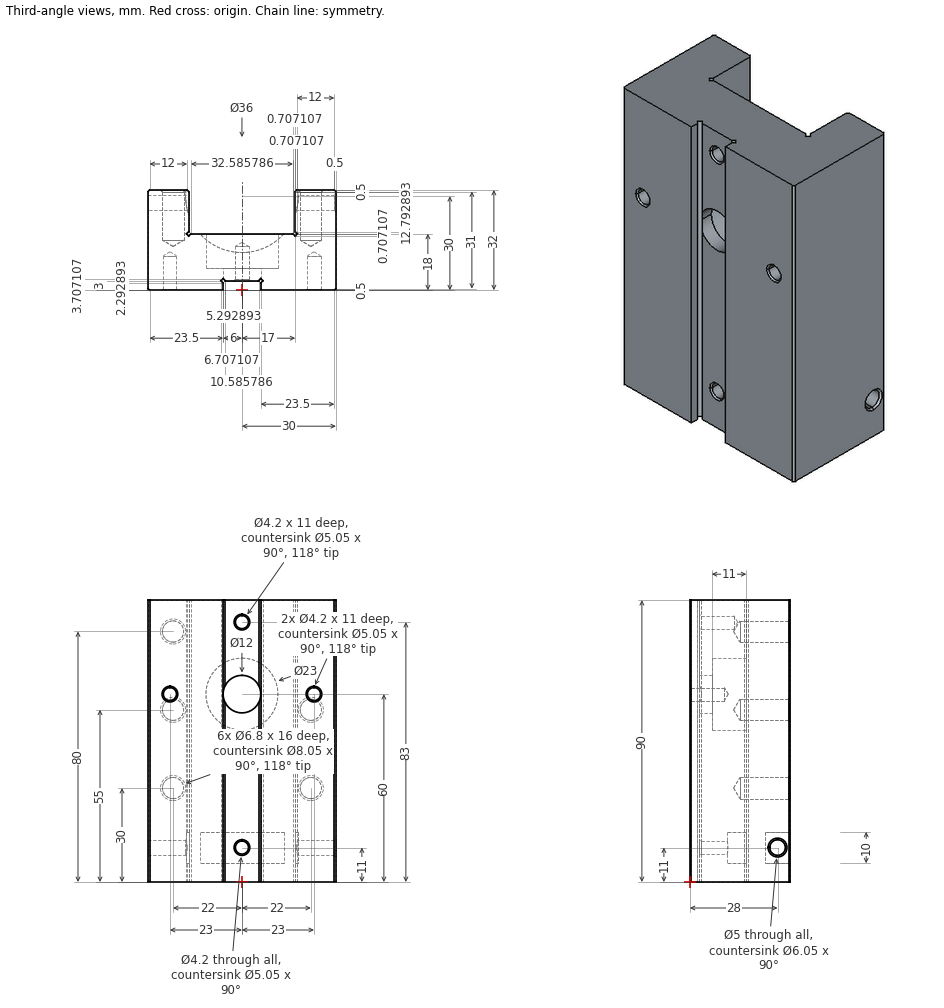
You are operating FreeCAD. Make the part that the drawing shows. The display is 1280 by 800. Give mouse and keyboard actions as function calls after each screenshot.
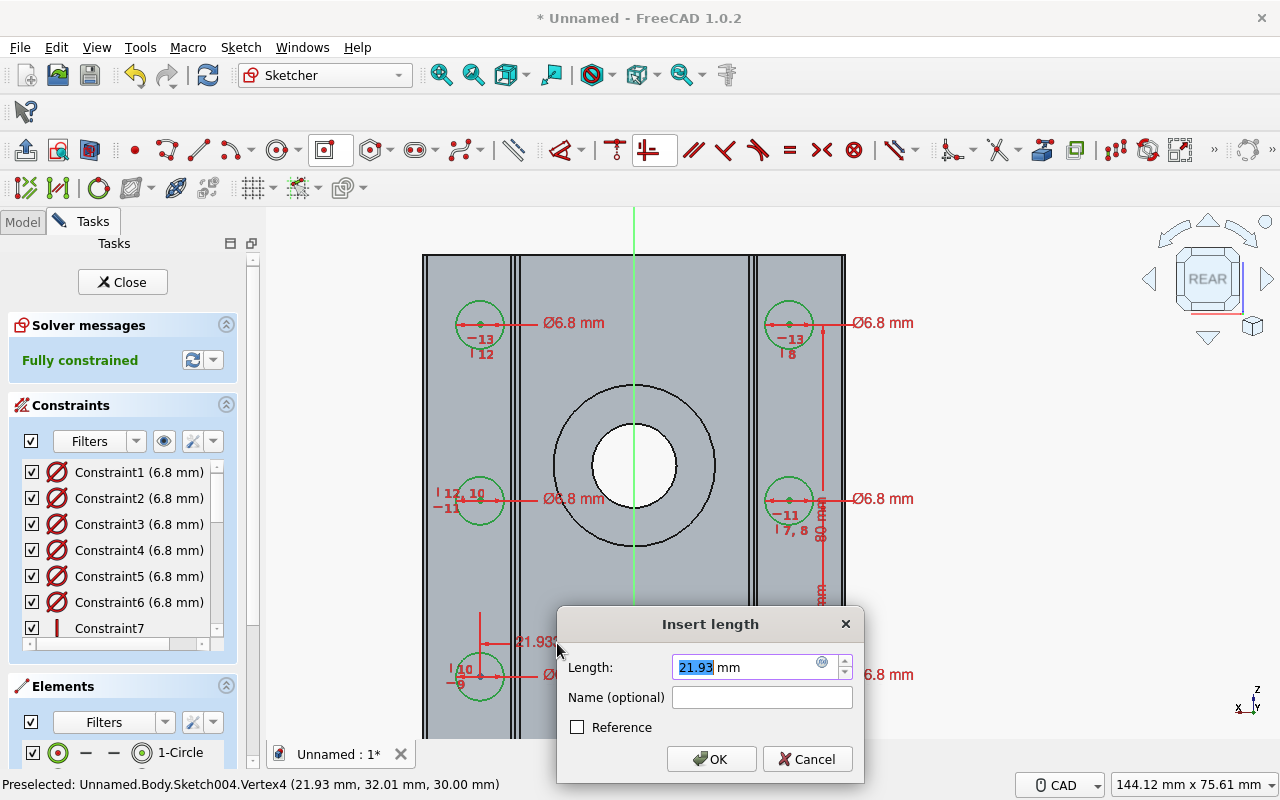
text(22)
key(Return)
key(Escape)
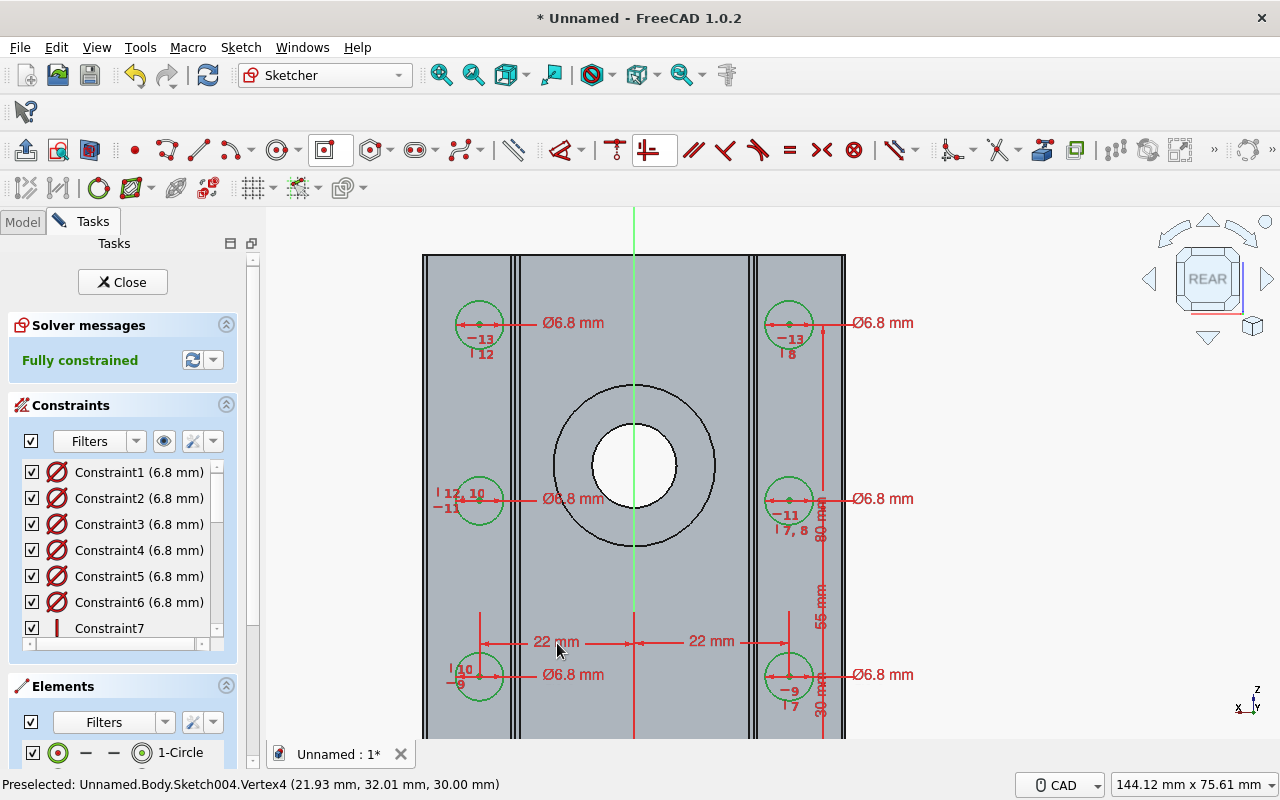
click(123, 282)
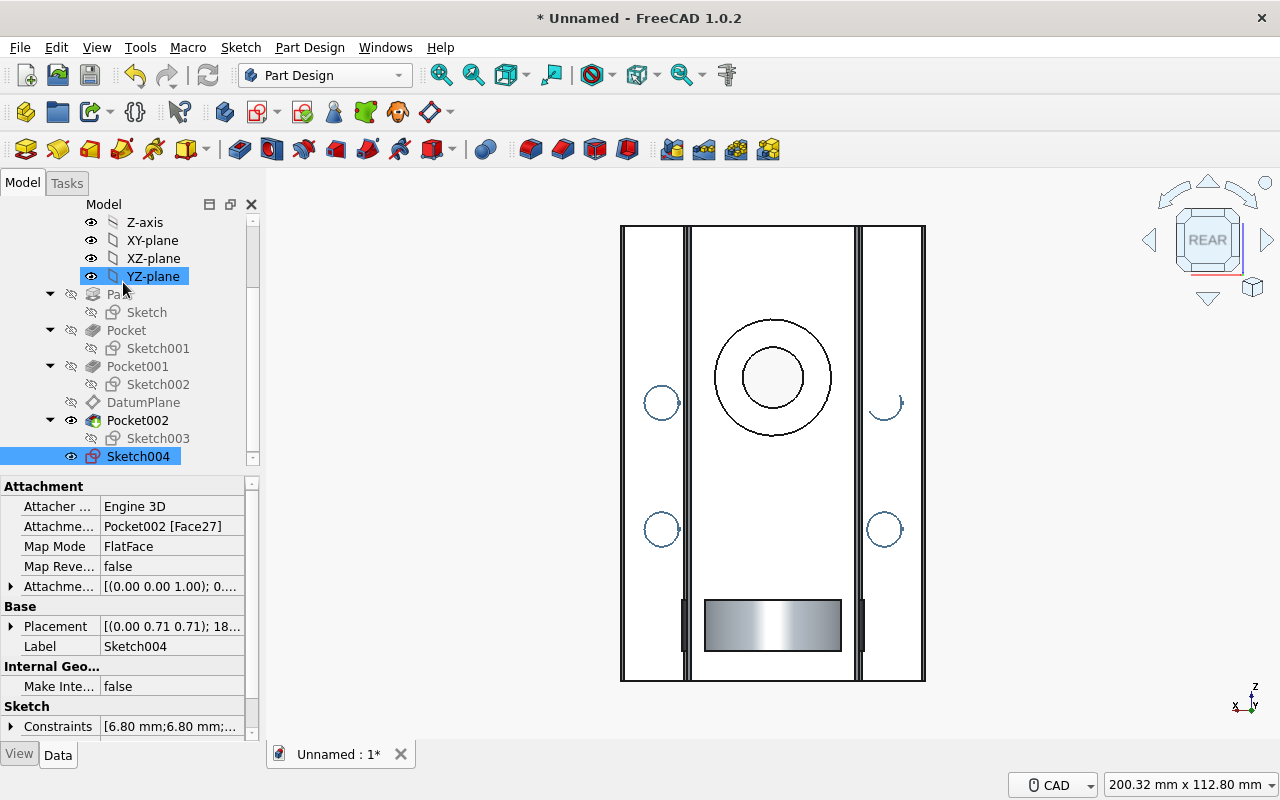
click(272, 150)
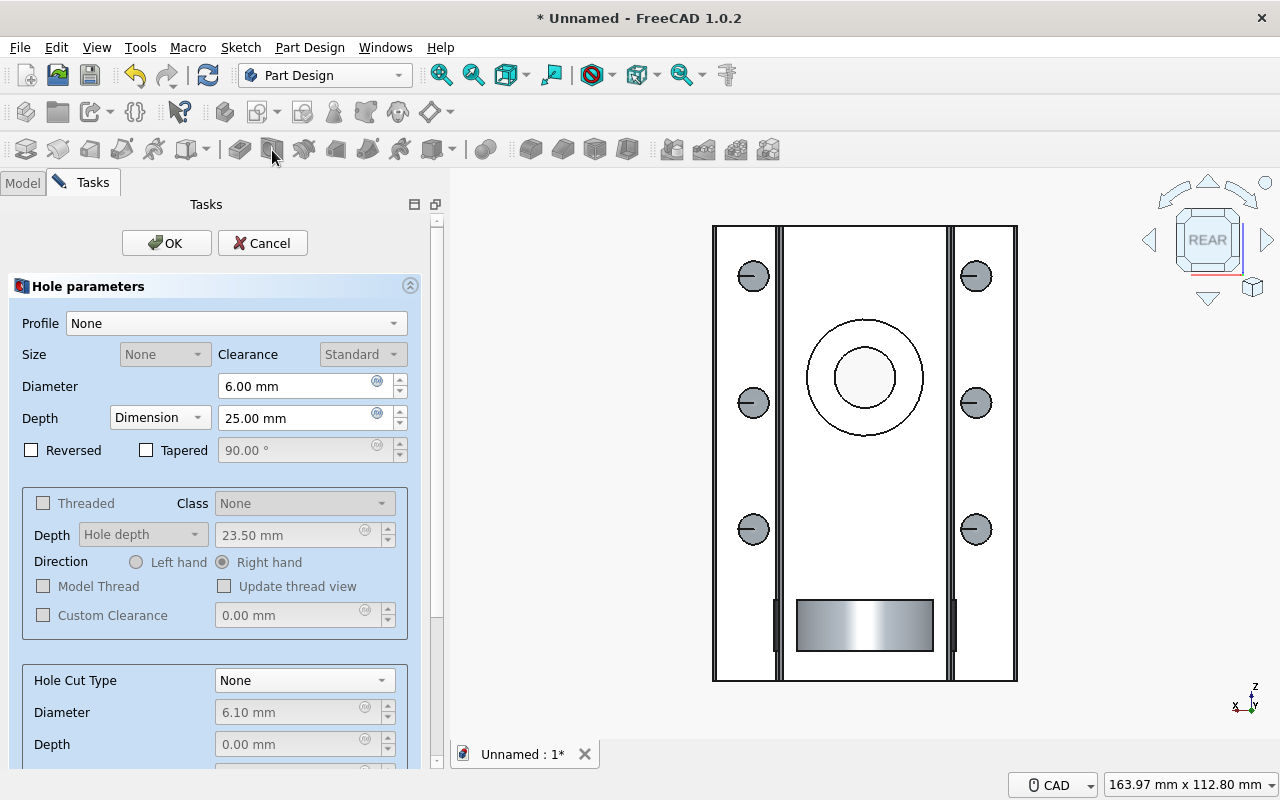
triple_click(305, 386)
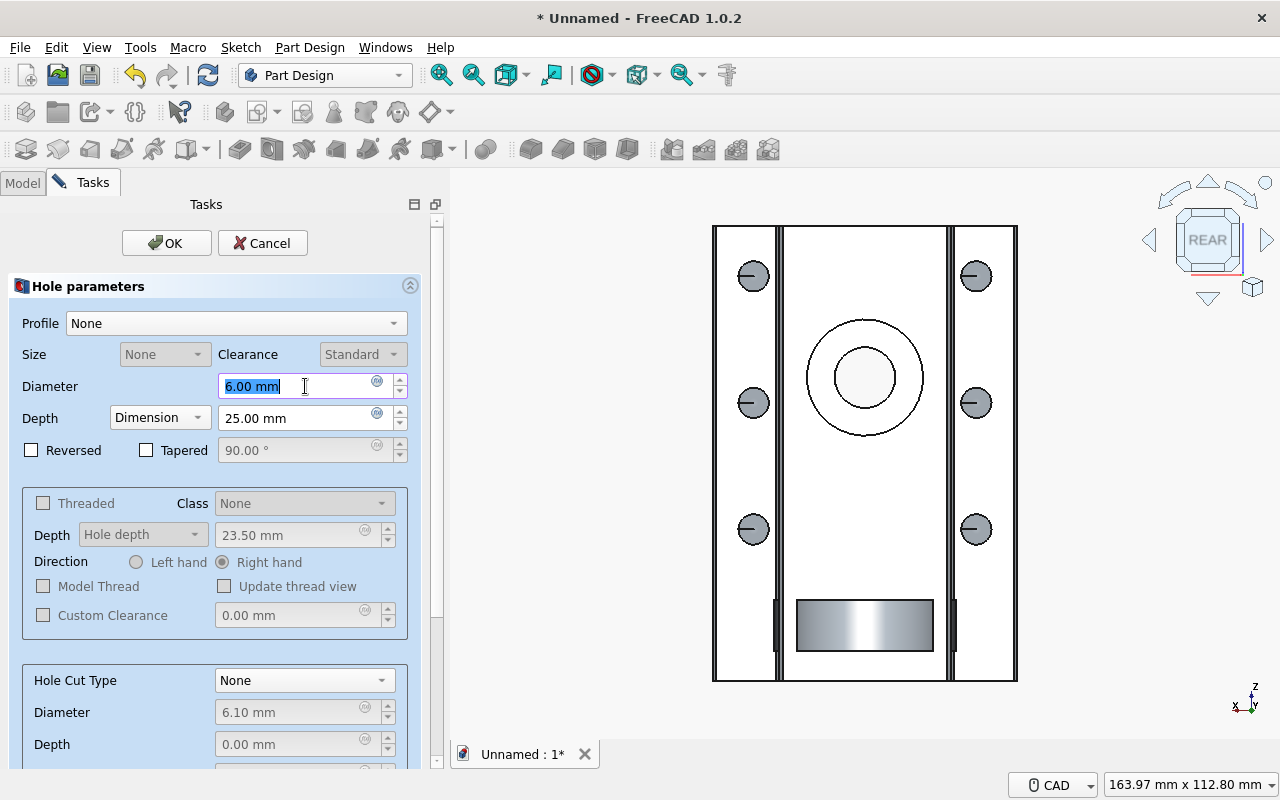
text(6.8)
key(Tab)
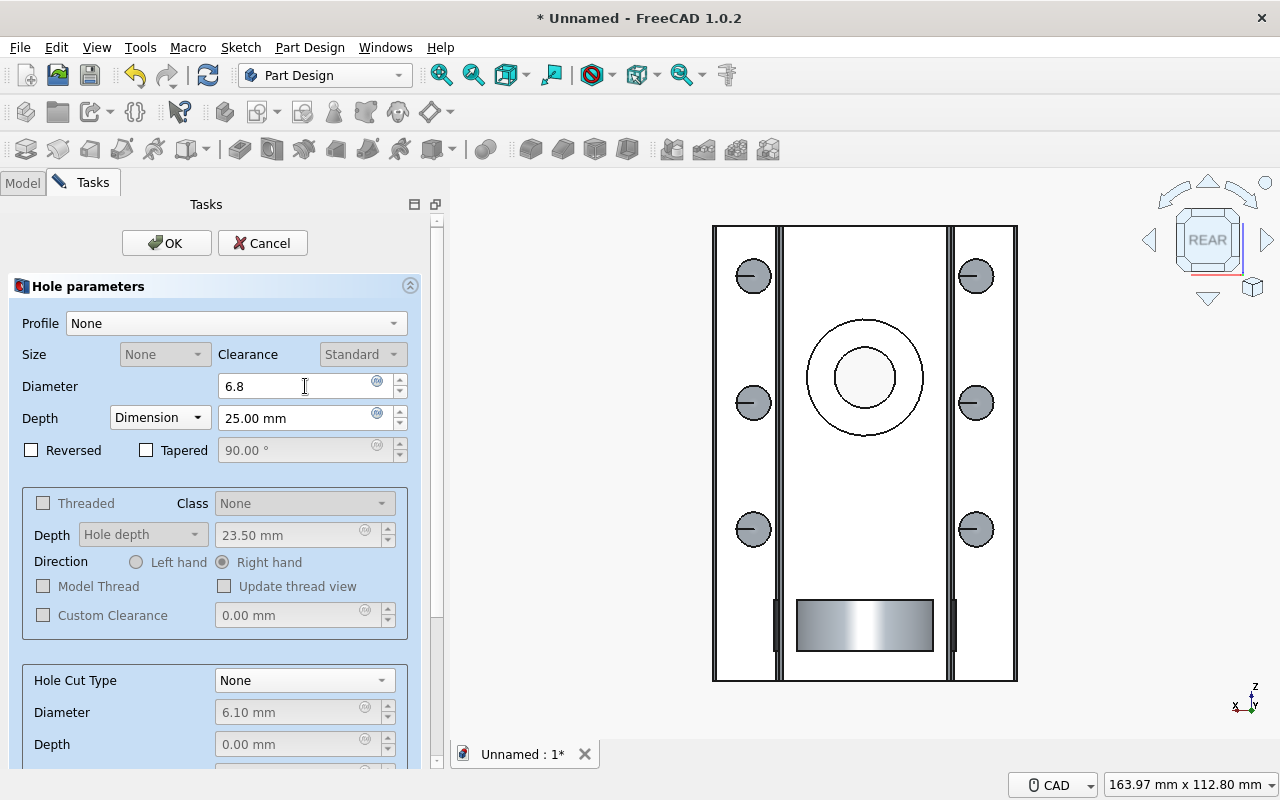
triple_click(305, 418)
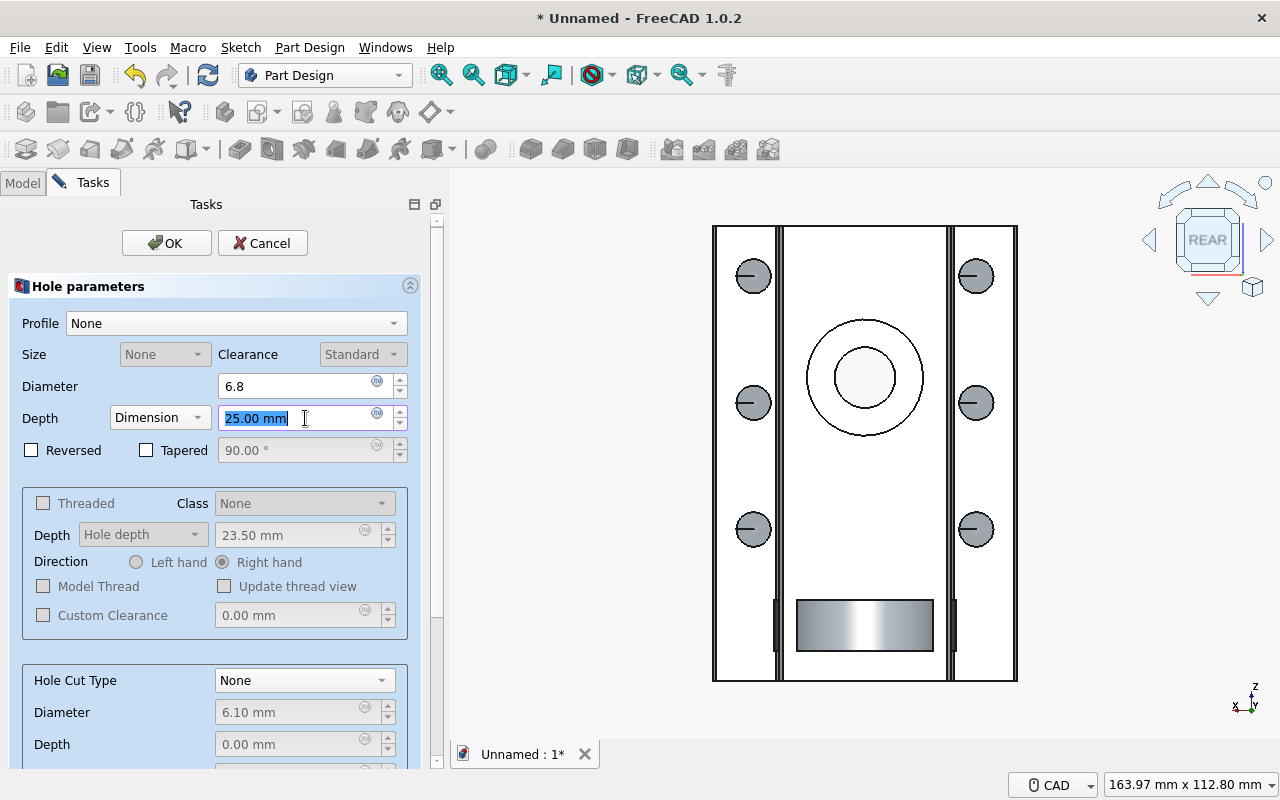
text(16)
key(Tab)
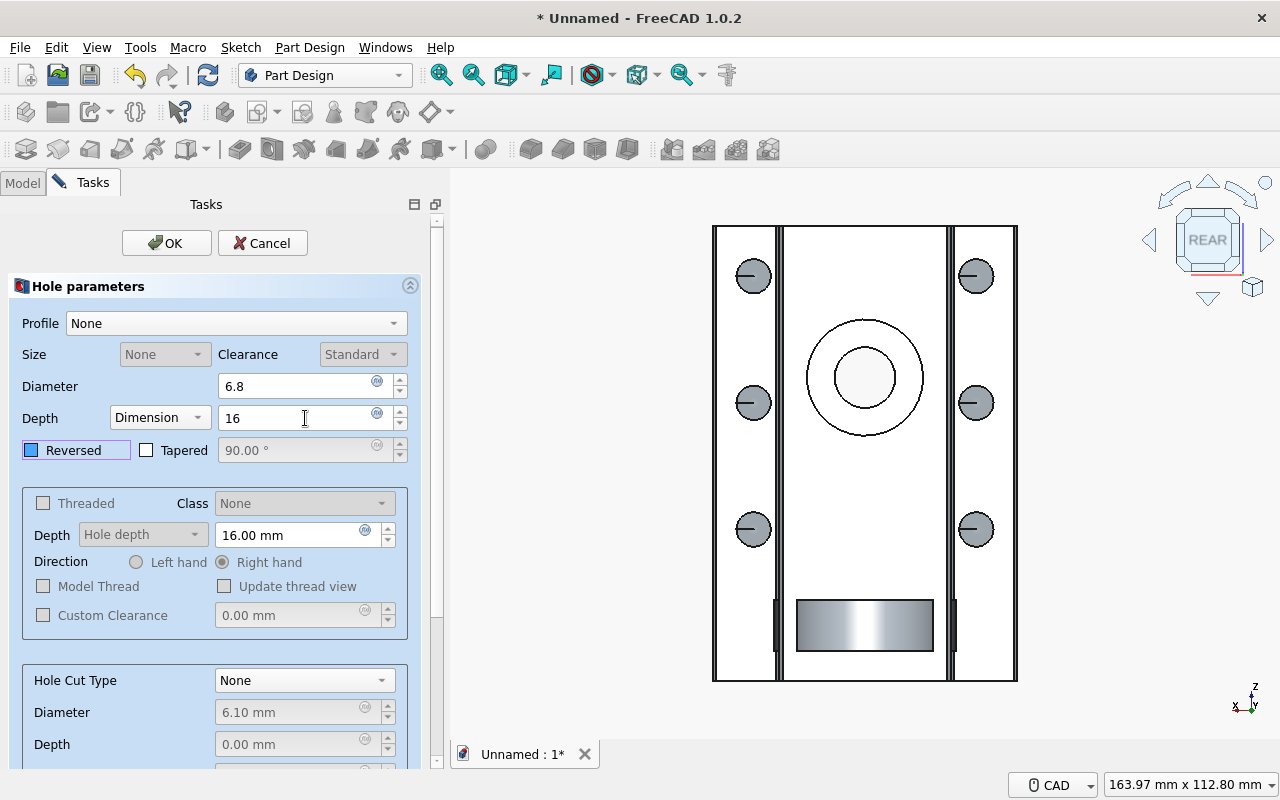
click(306, 680)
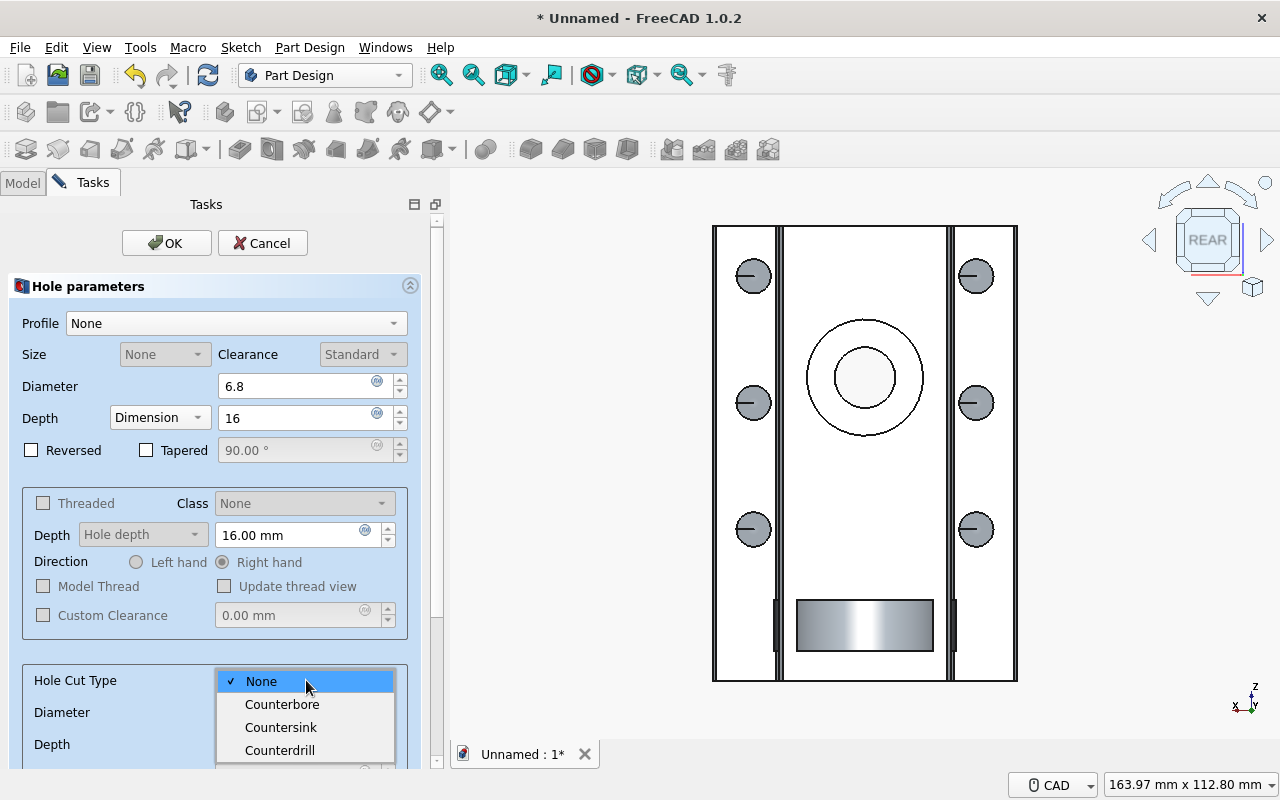
click(304, 728)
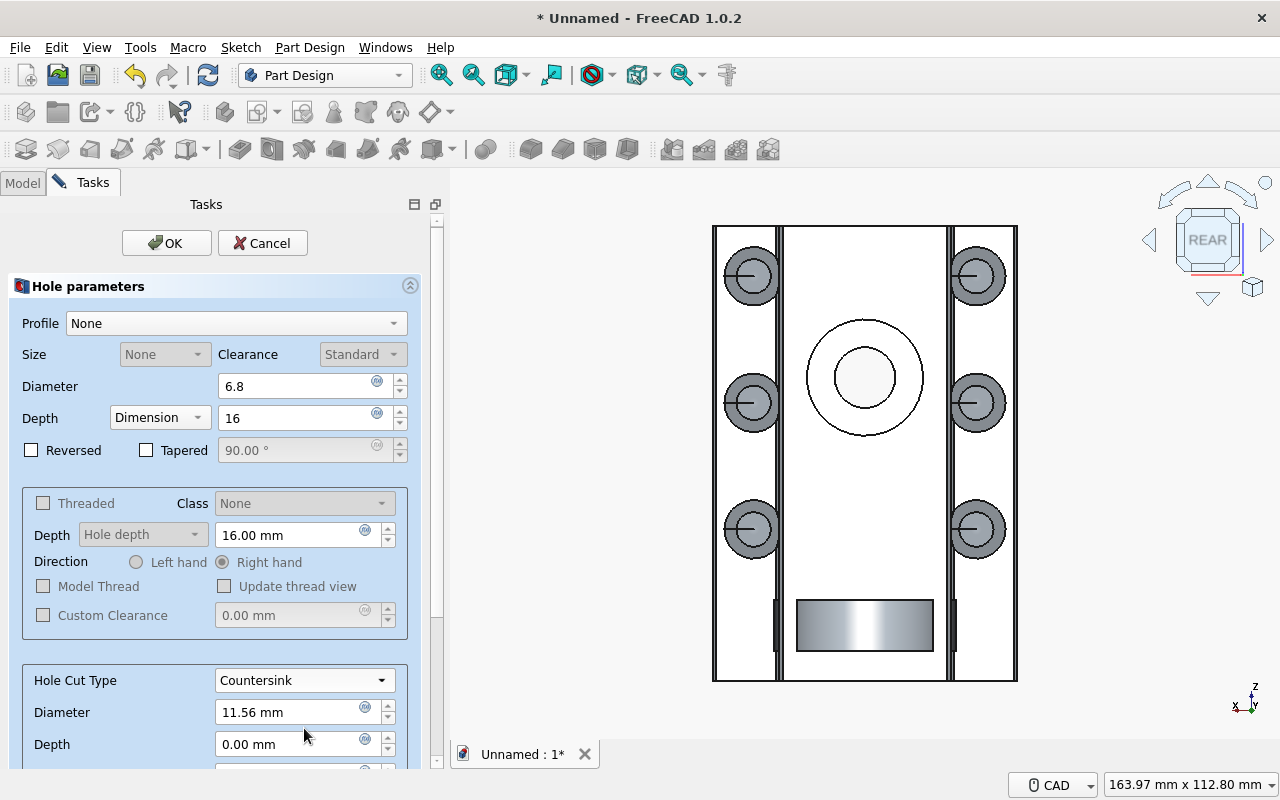
triple_click(298, 712)